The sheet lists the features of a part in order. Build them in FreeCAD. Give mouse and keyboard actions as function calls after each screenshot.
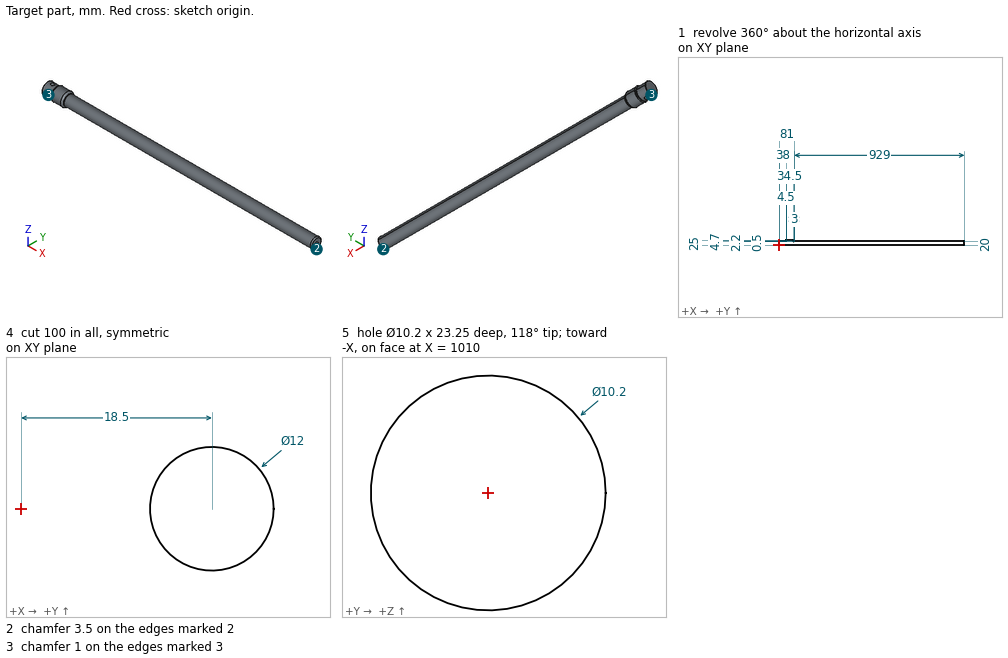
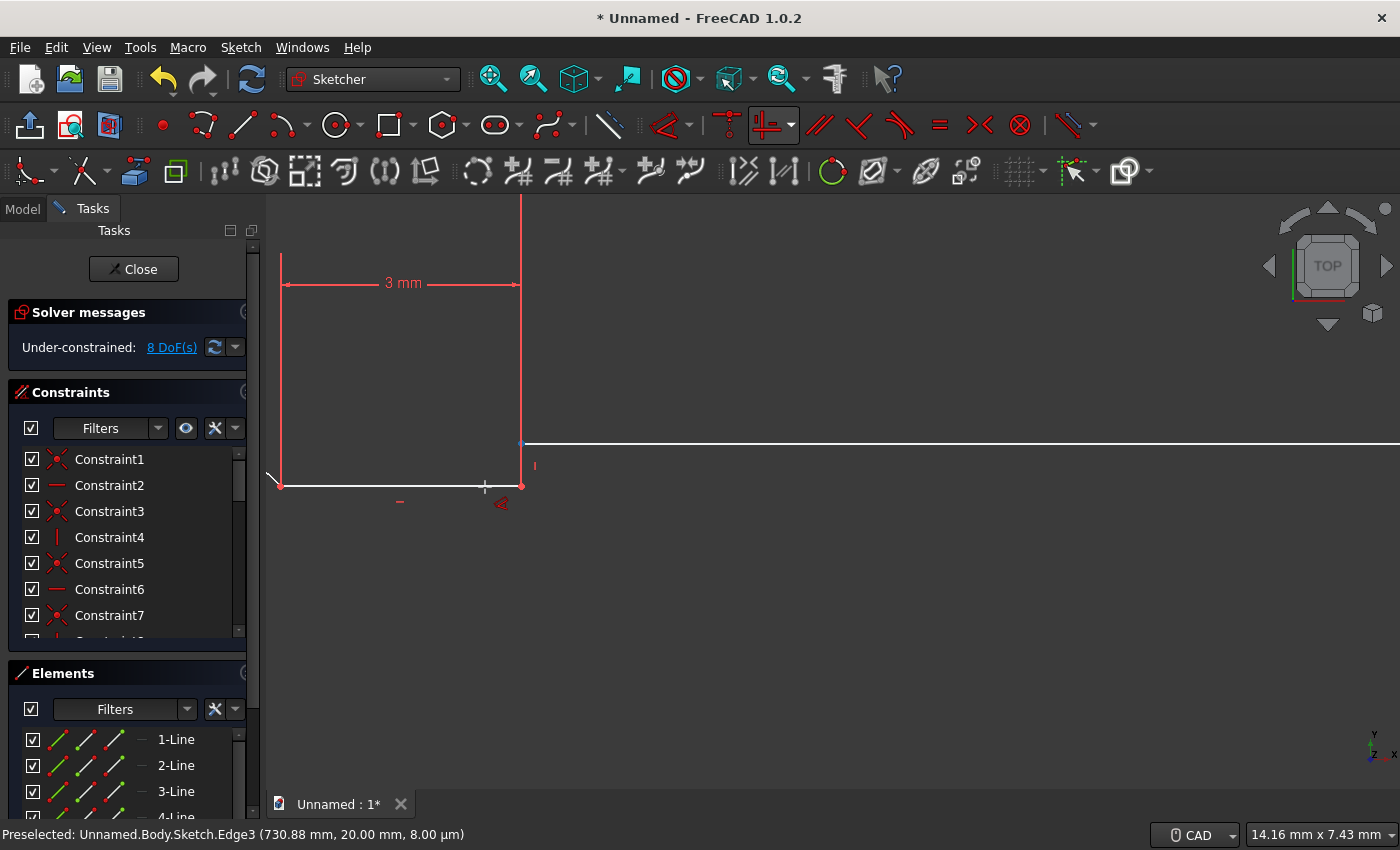
click(521, 465)
click(487, 465)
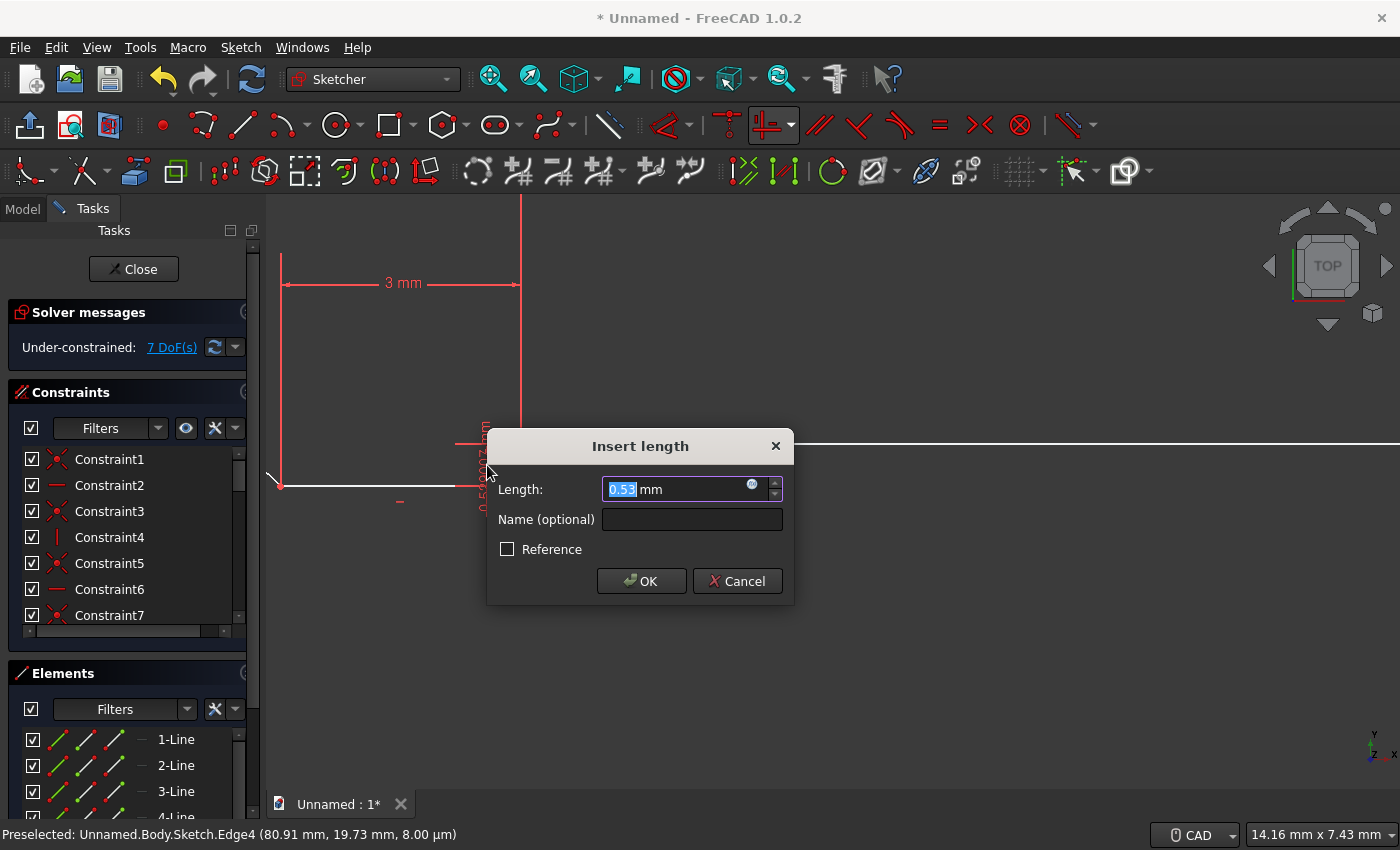
text(0.5)
key(Return)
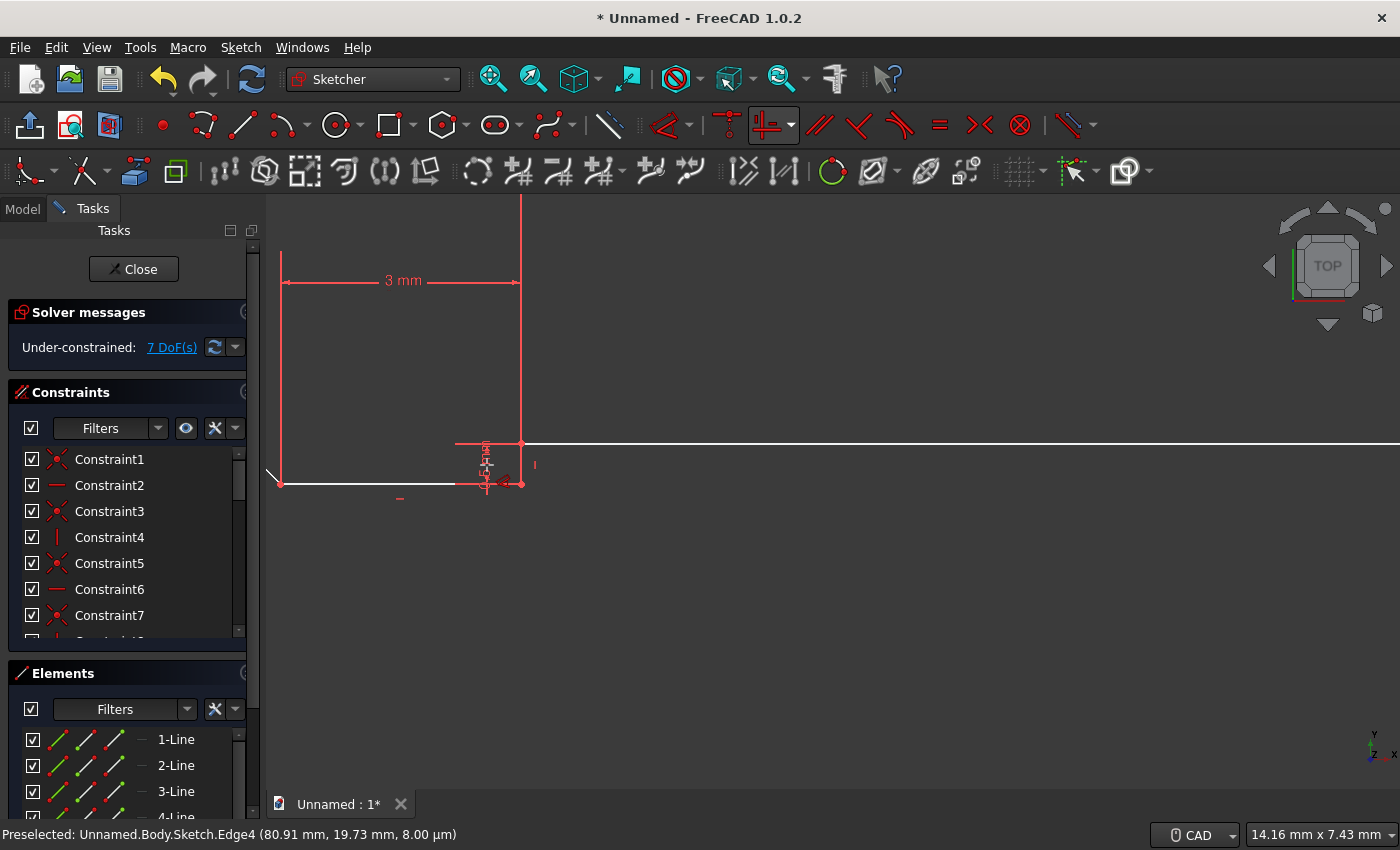
scroll(764, 492, down, 15)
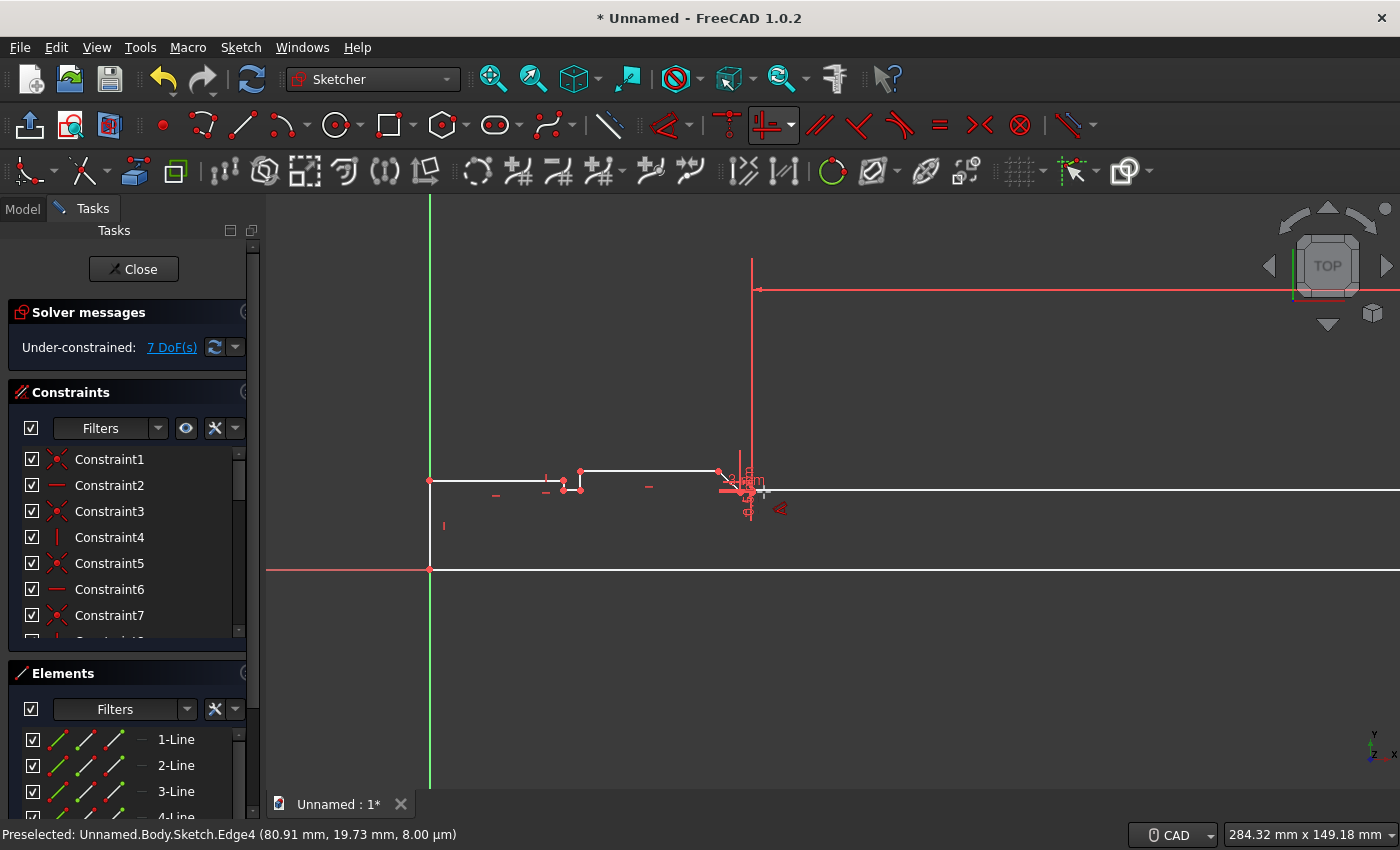
scroll(432, 486, down, 9)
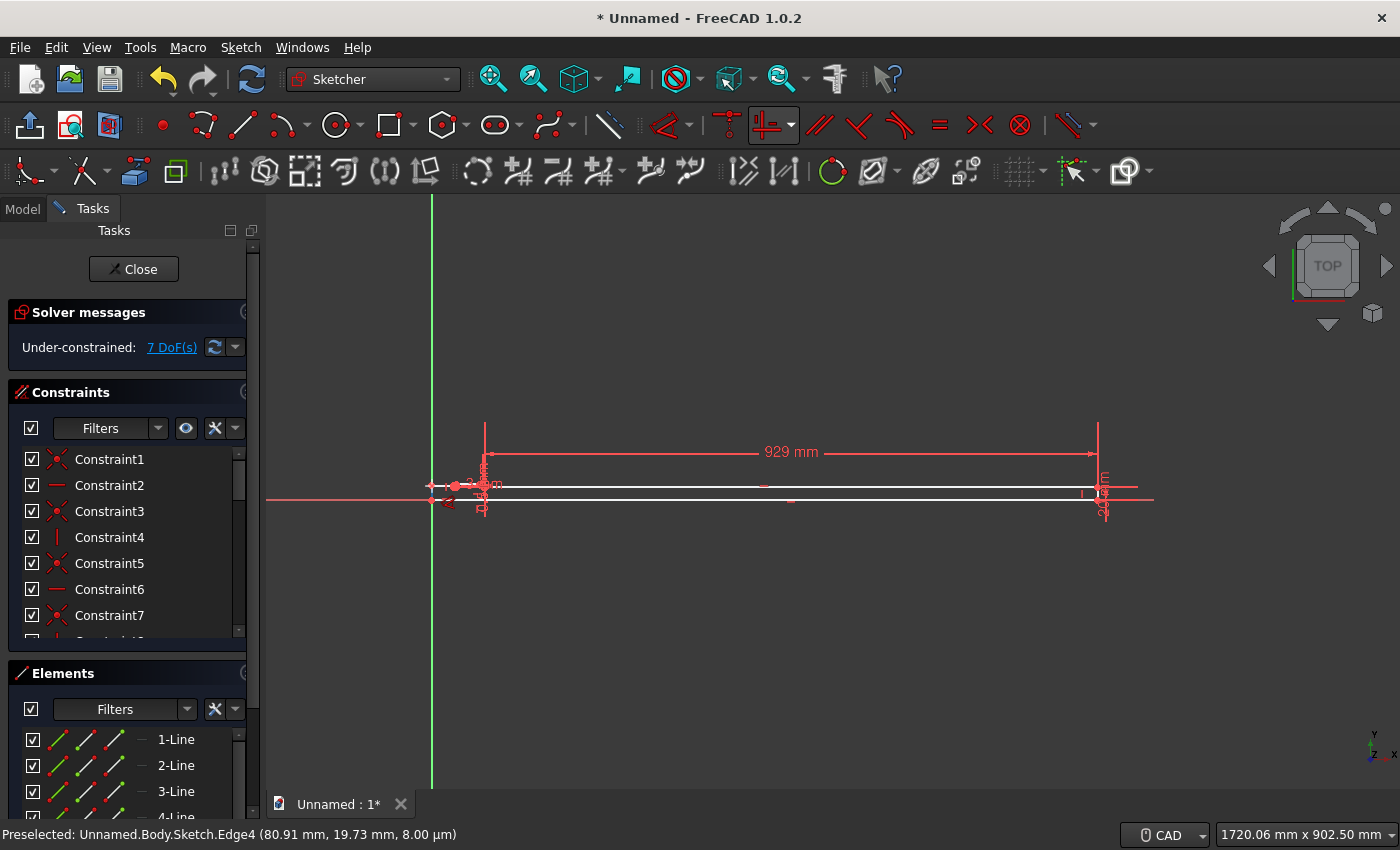
scroll(457, 485, up, 14)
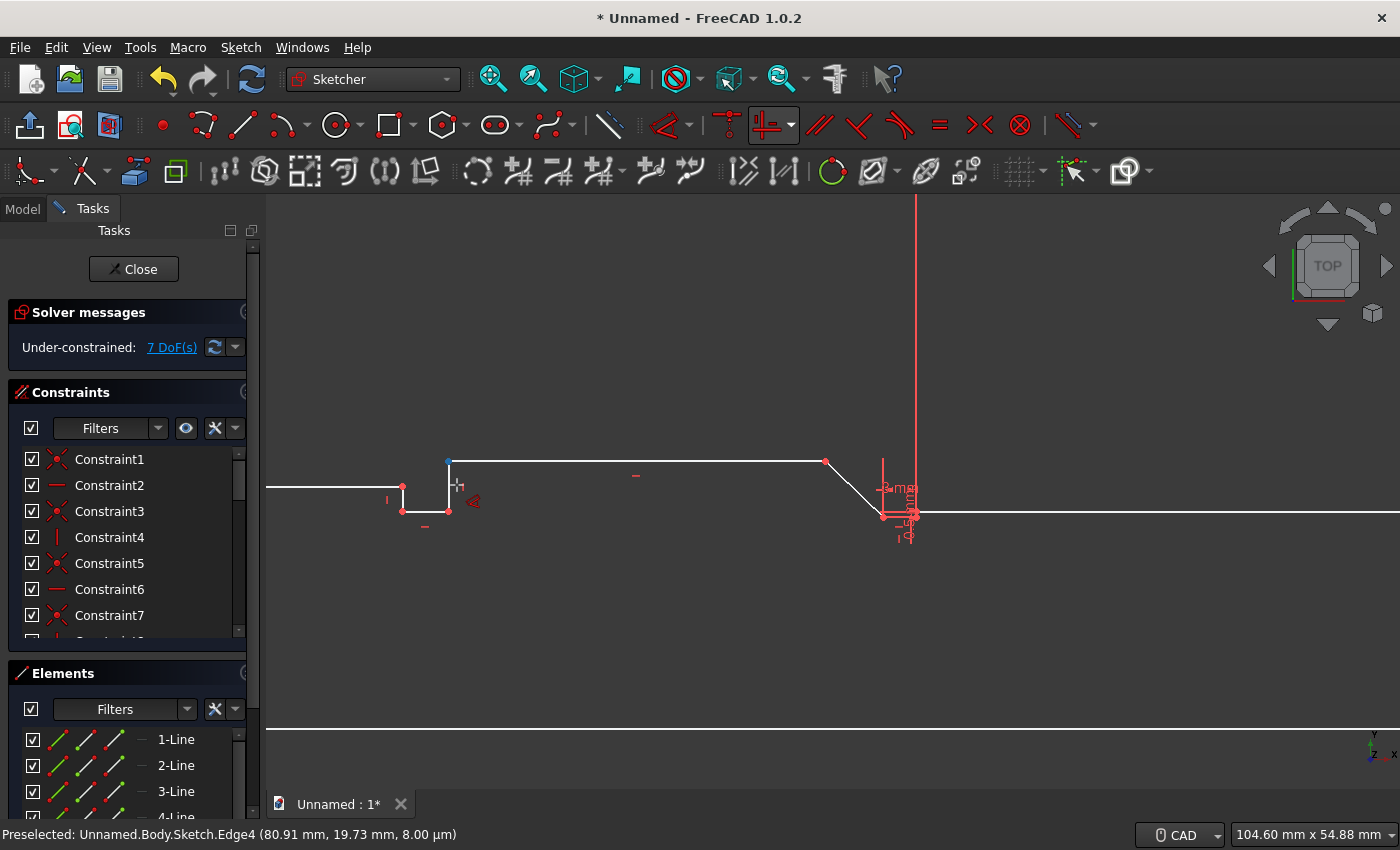
click(449, 476)
click(415, 475)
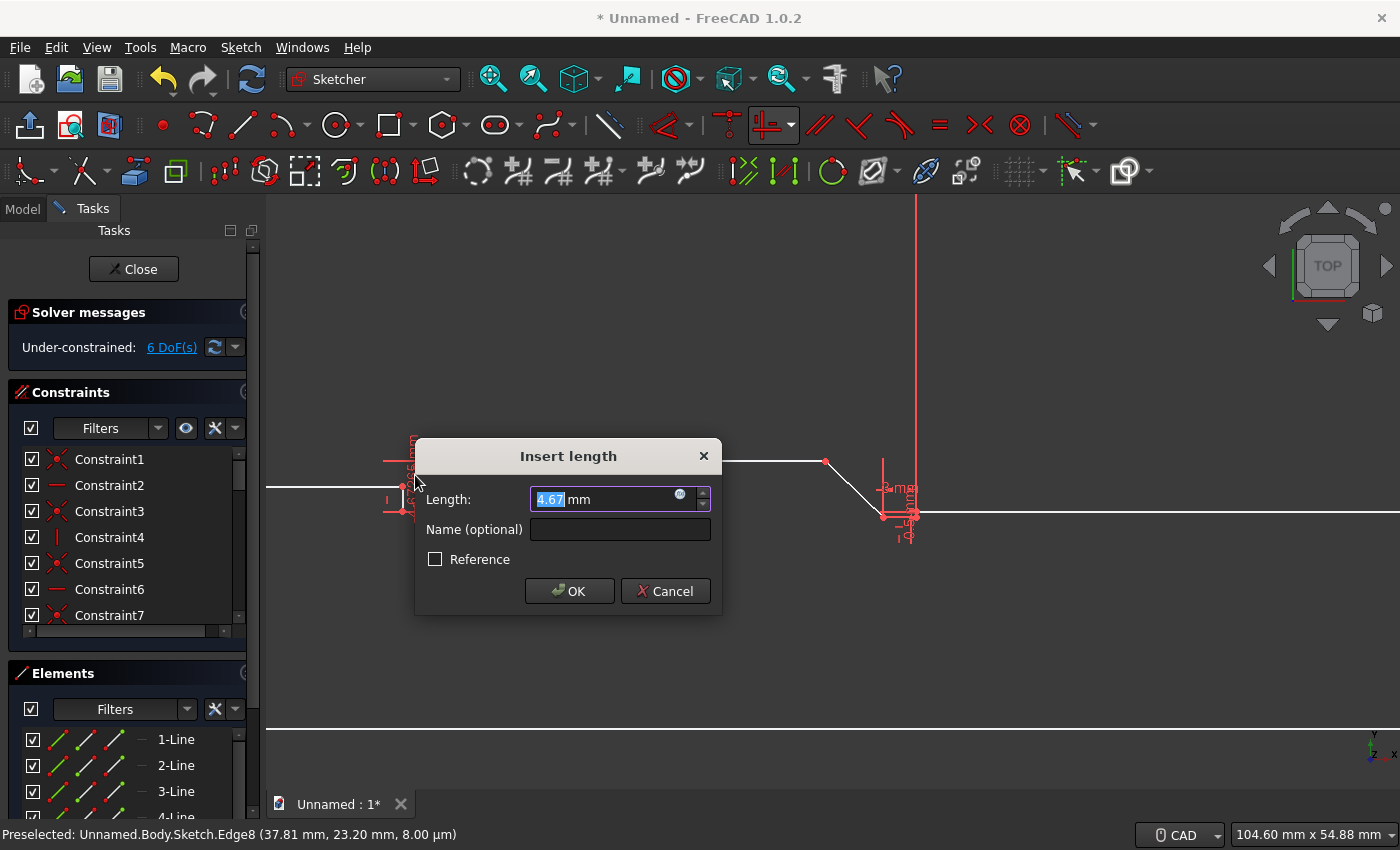
text(4.7)
key(Return)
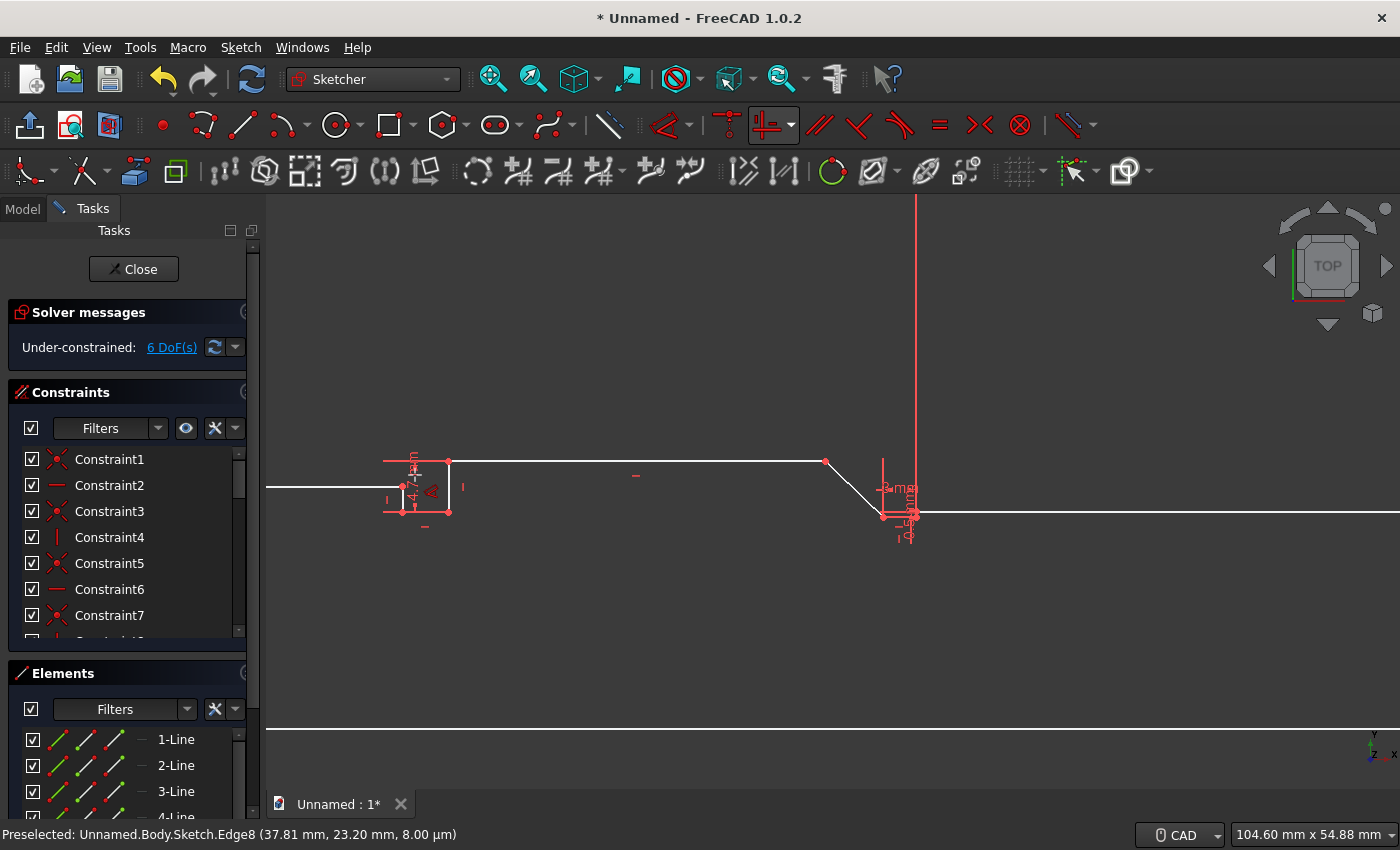
click(435, 512)
click(426, 546)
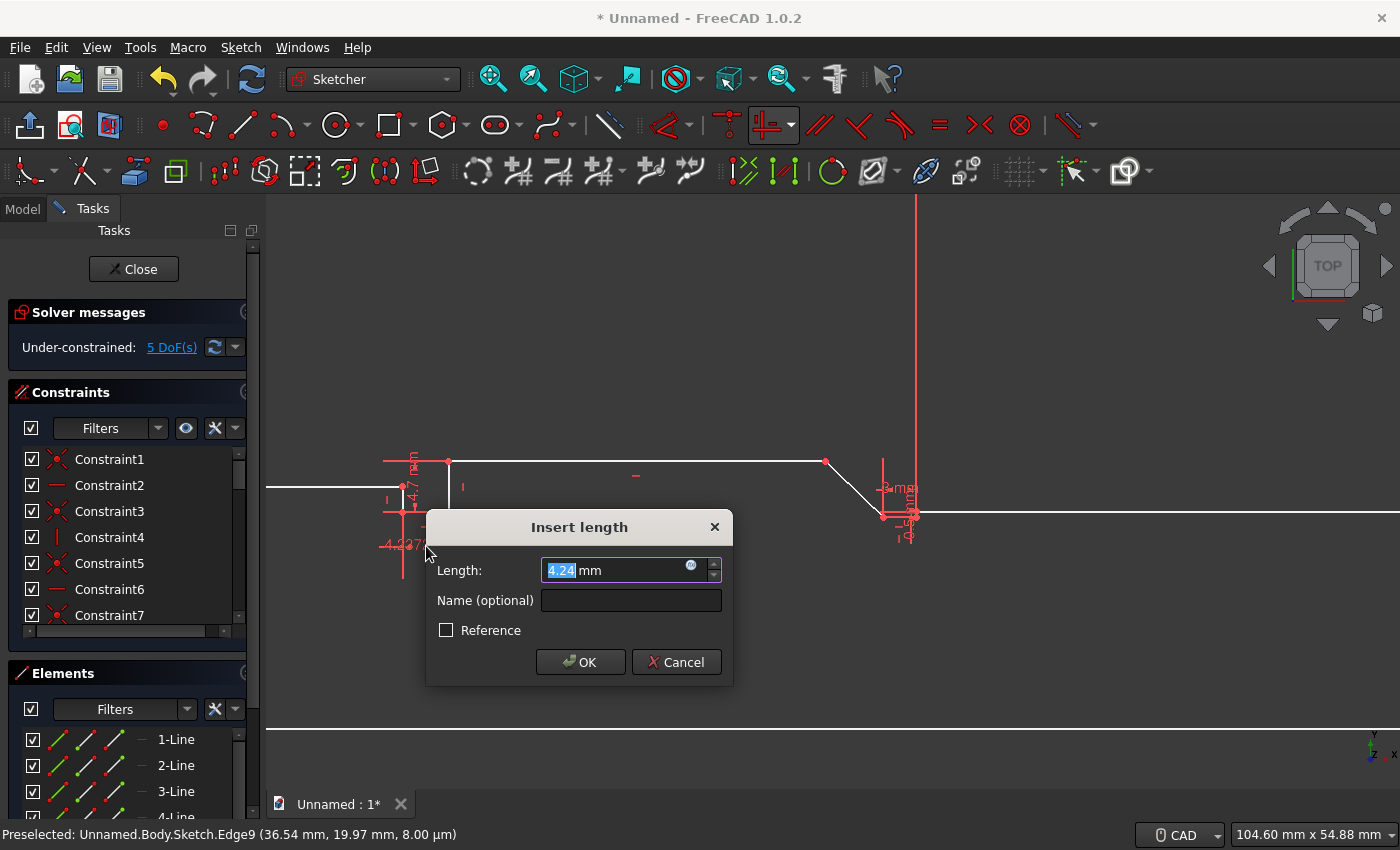
text(4.5)
key(Return)